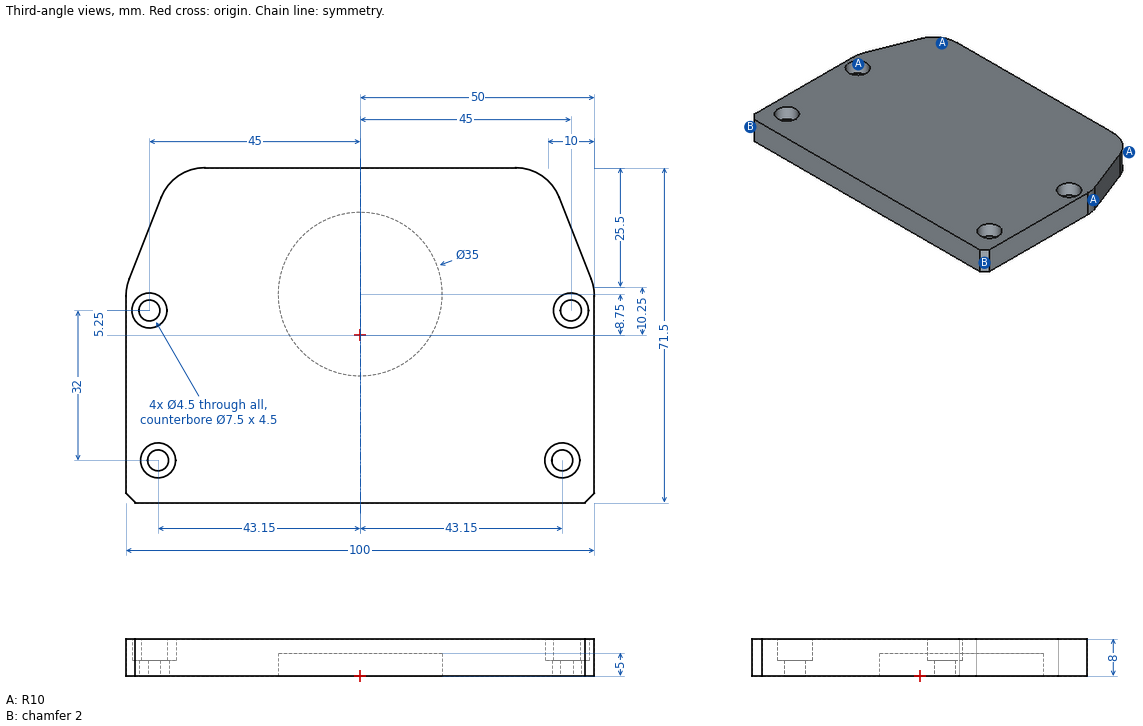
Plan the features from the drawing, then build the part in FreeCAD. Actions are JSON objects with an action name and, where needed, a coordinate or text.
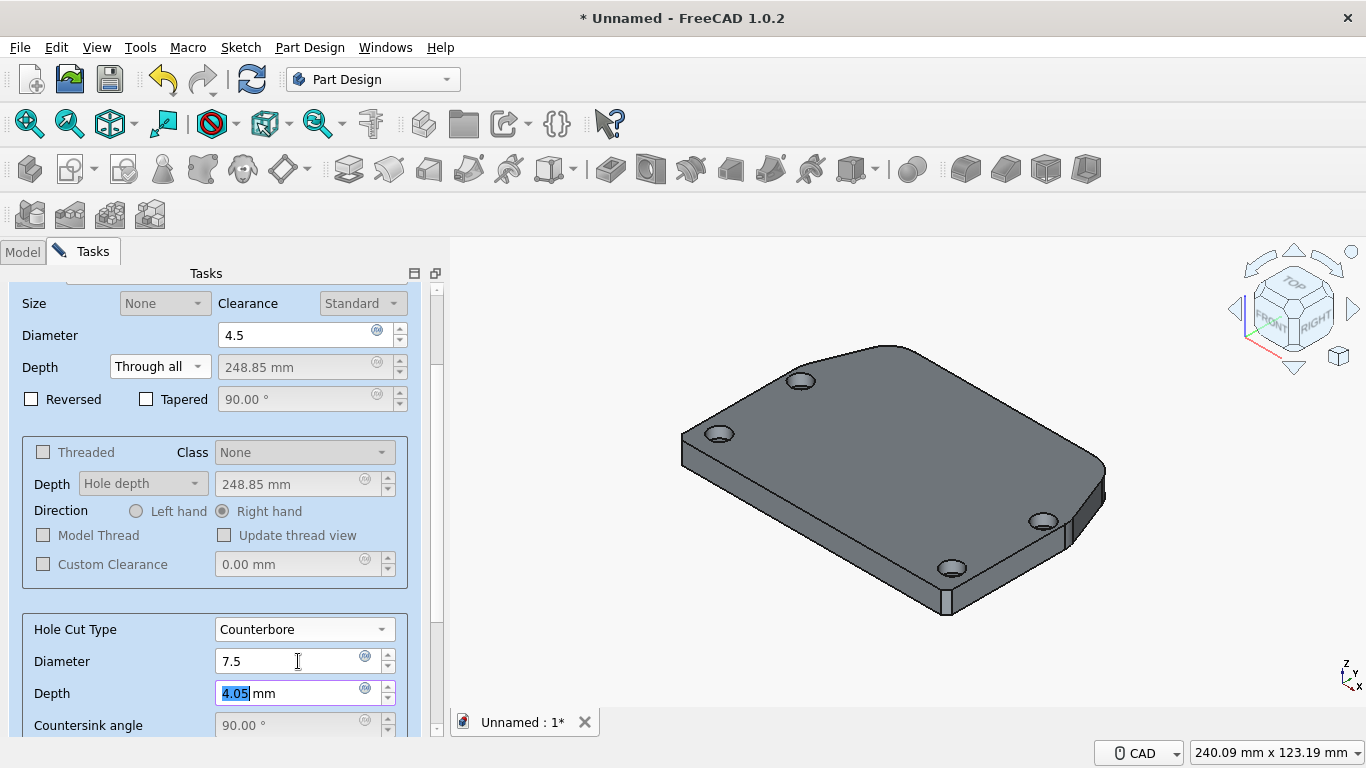
{"action": "type", "text": "4.5"}
{"action": "key", "text": "Tab"}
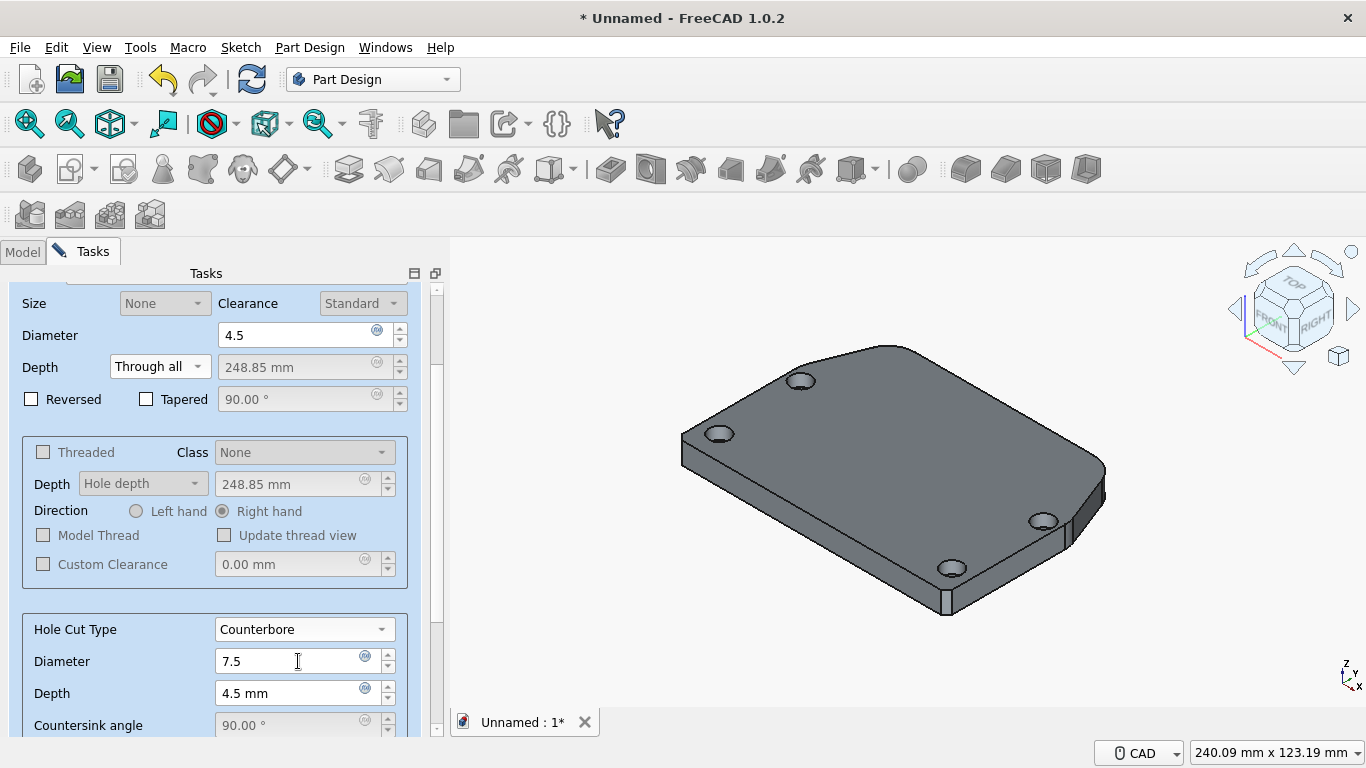
{"action": "scroll", "coordinate": [437, 510], "scroll_direction": "up", "scroll_amount": 3}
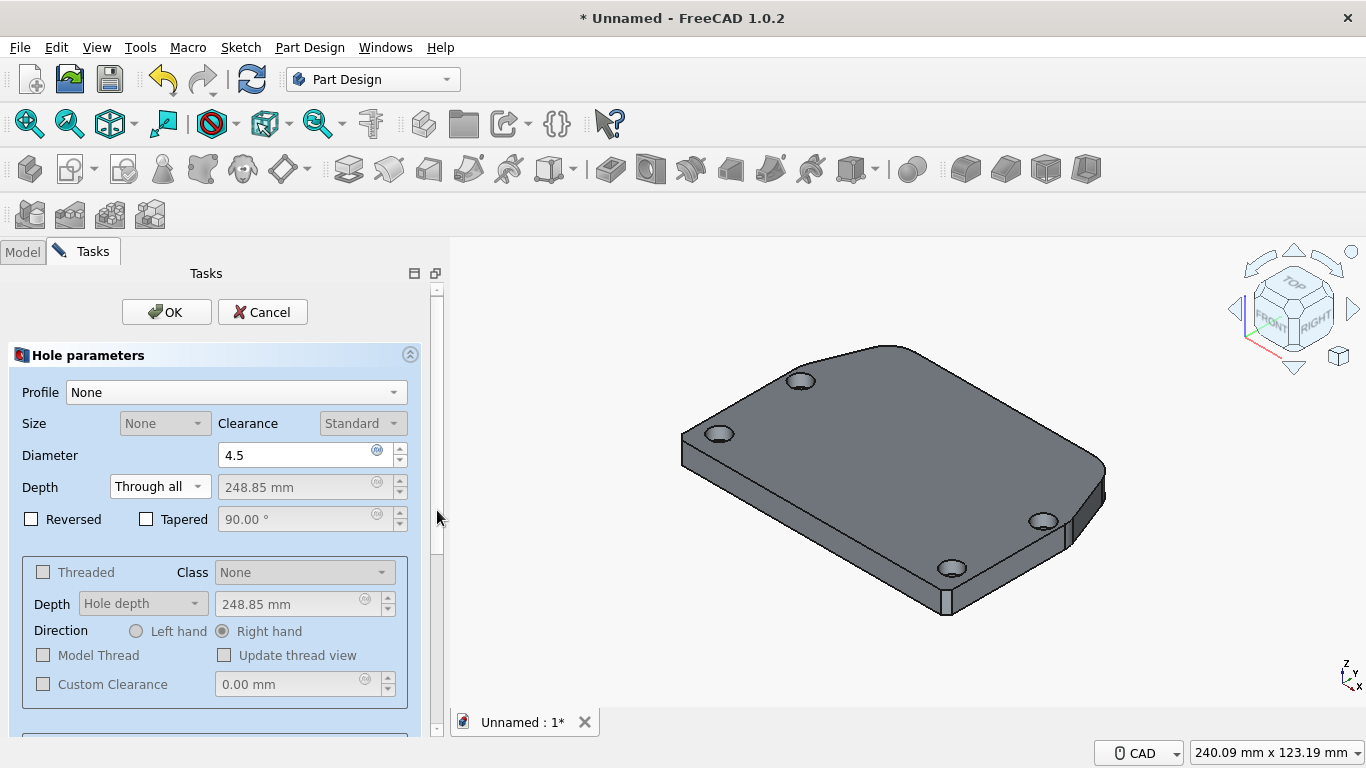
{"action": "left_click", "coordinate": [167, 312]}